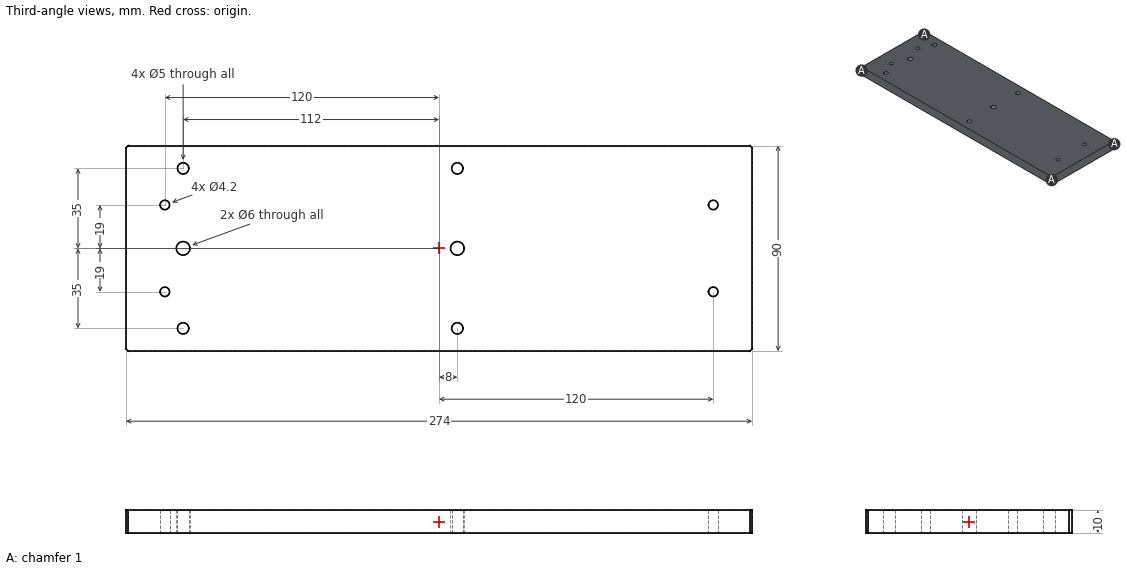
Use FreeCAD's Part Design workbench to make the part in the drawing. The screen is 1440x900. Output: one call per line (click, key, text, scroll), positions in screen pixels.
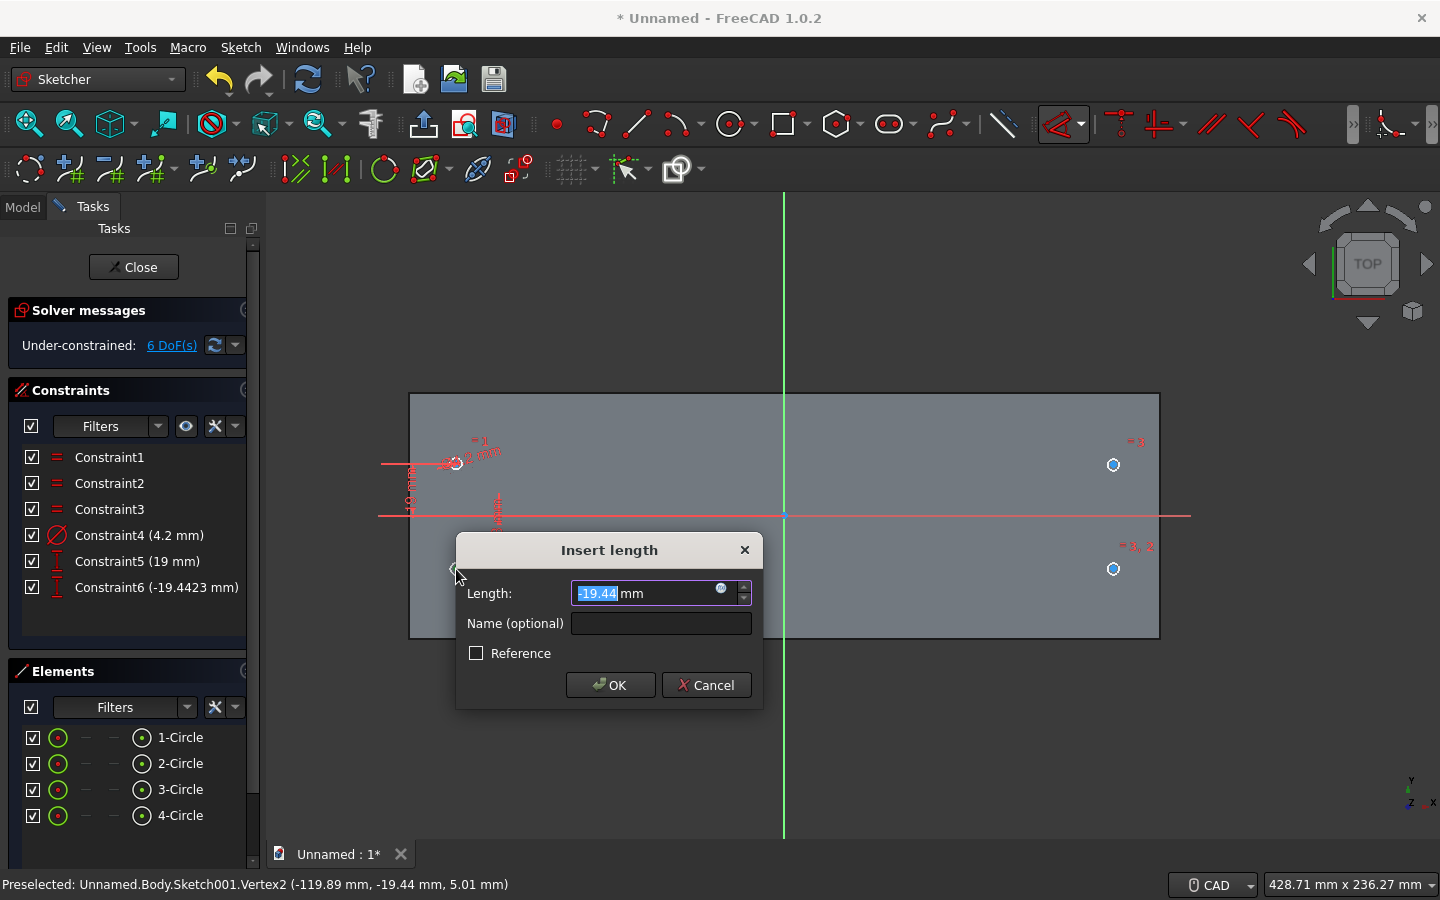
text(-19)
key(Return)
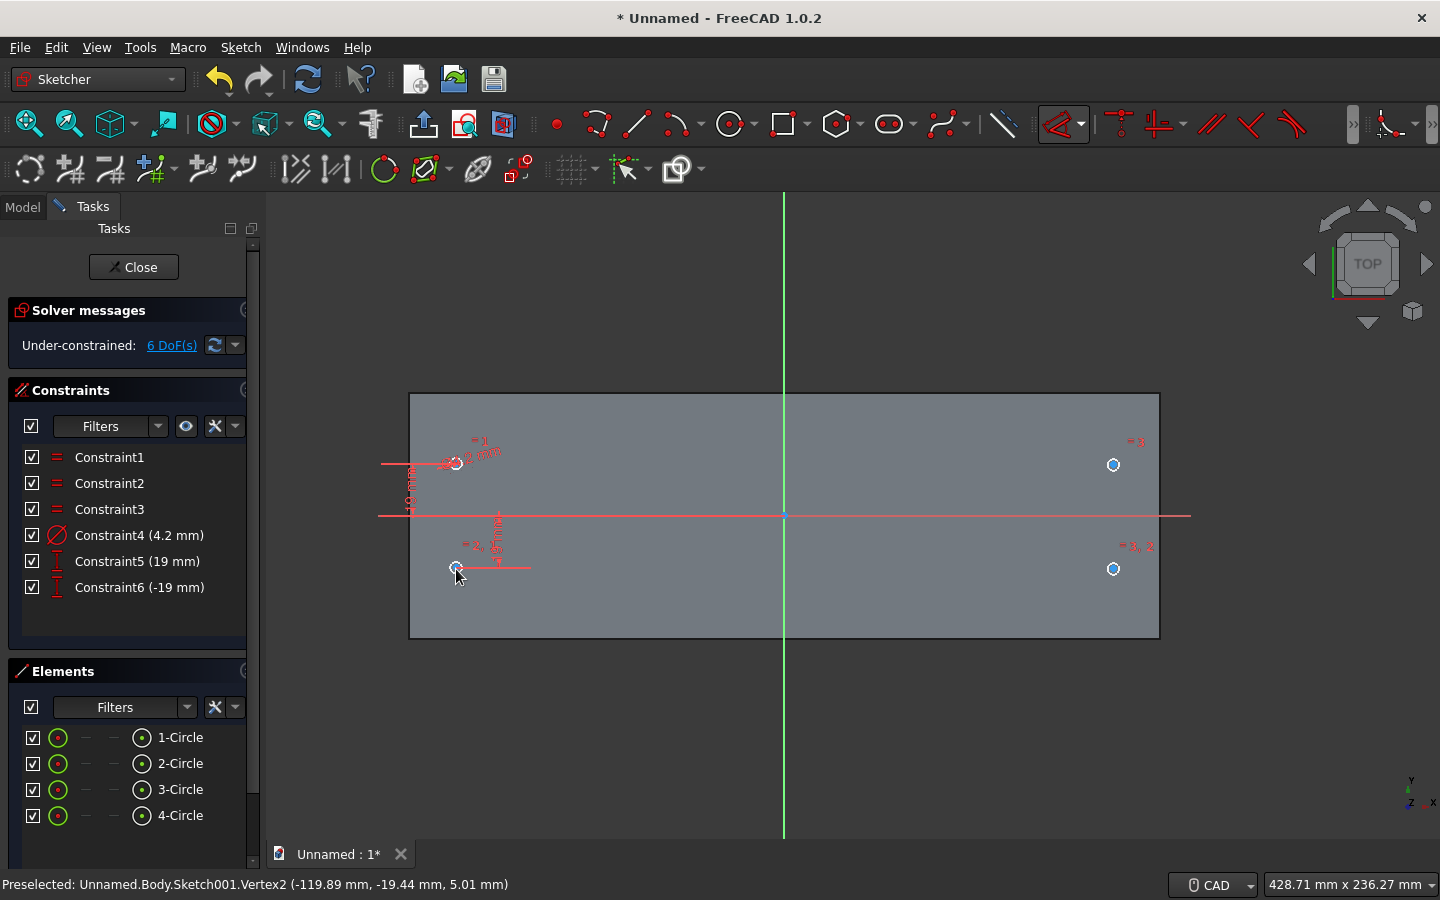
click(1113, 569)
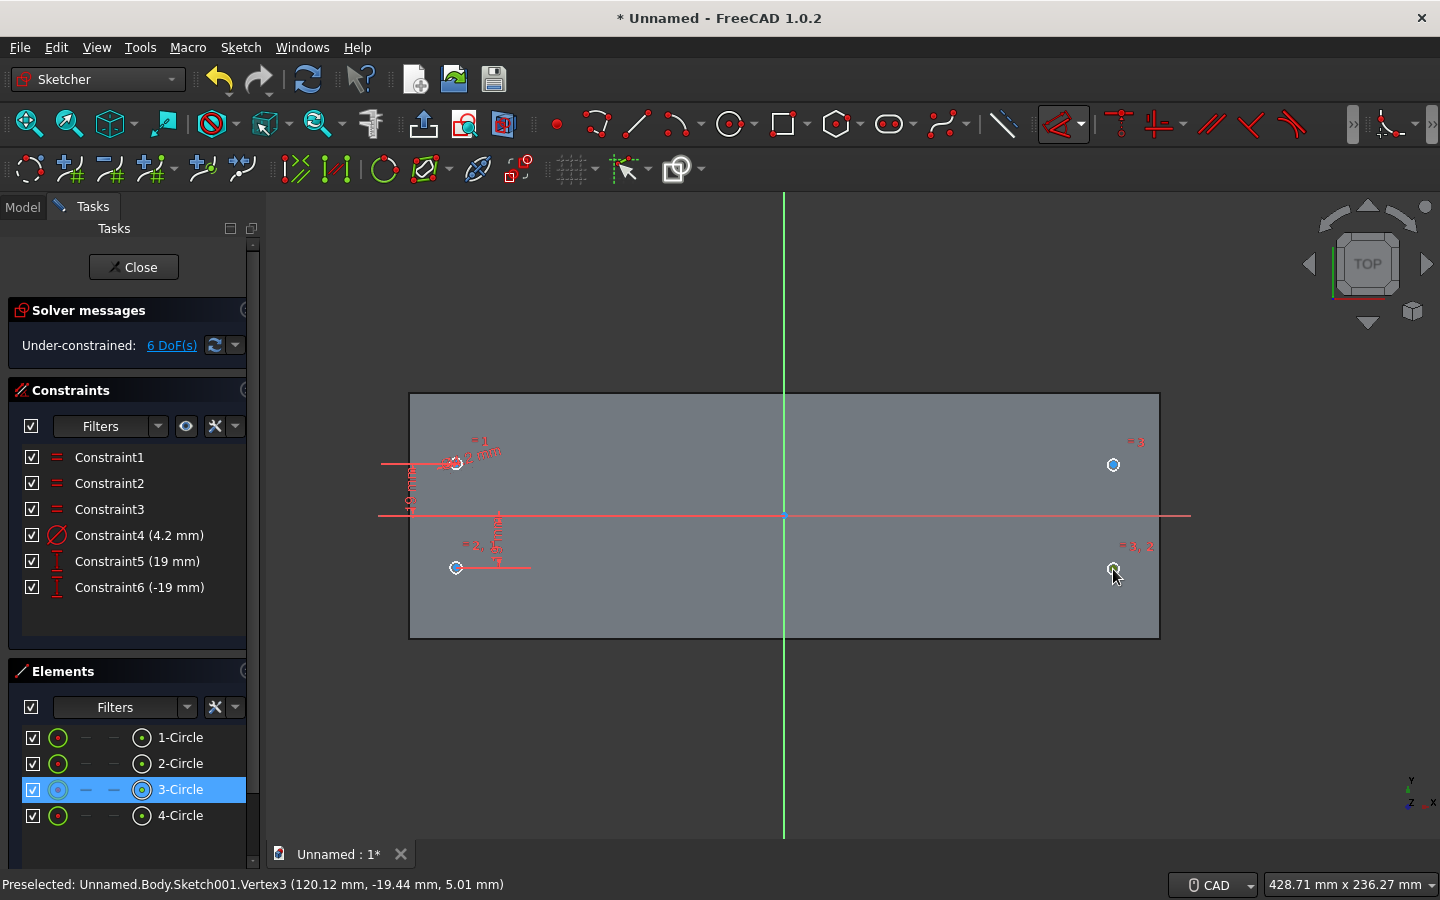
key(i)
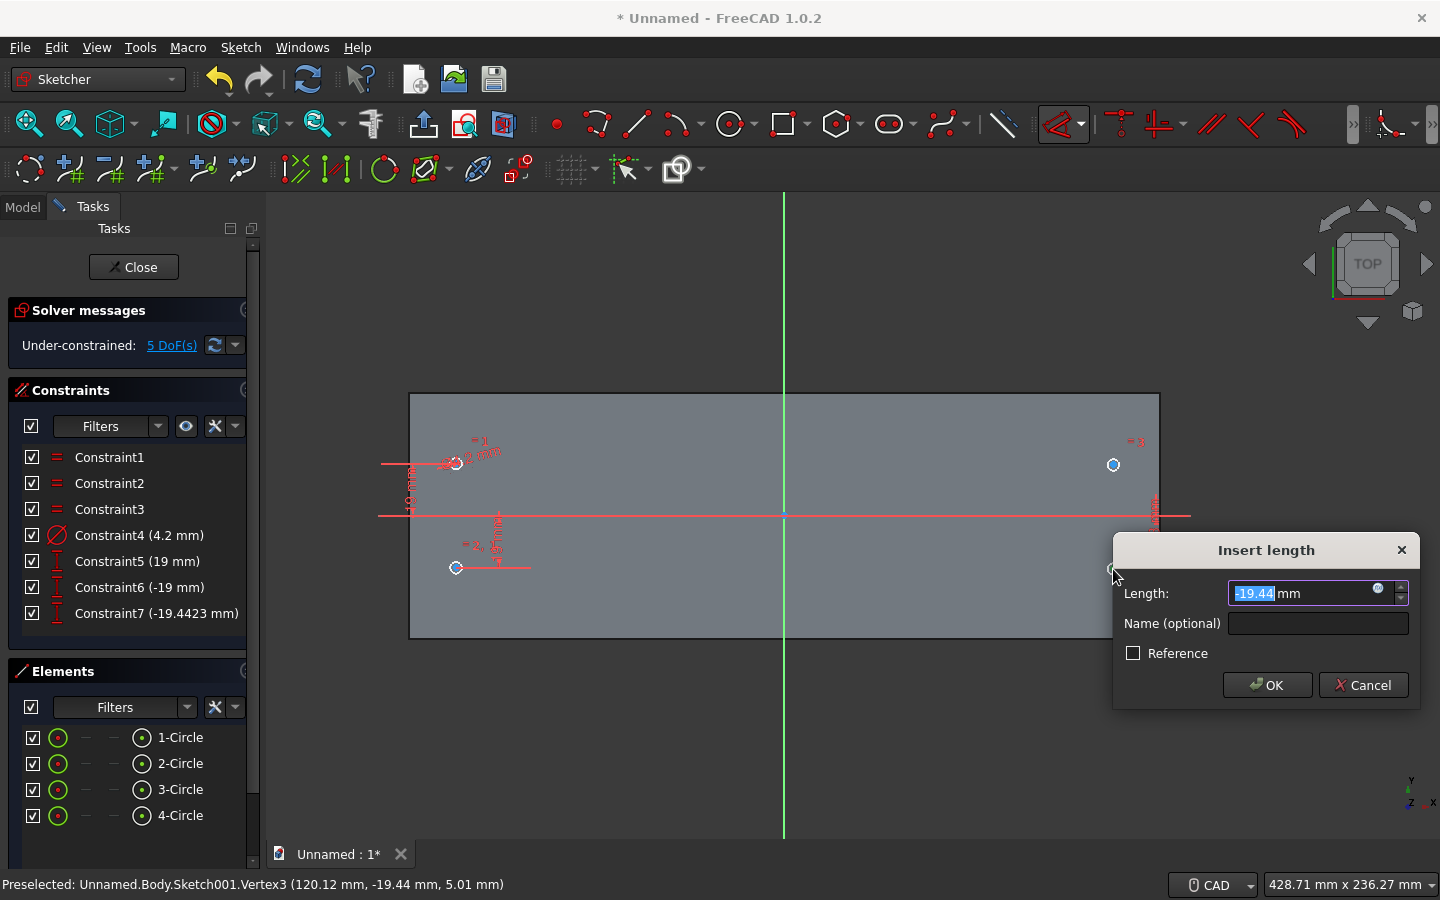
text(-19)
key(Return)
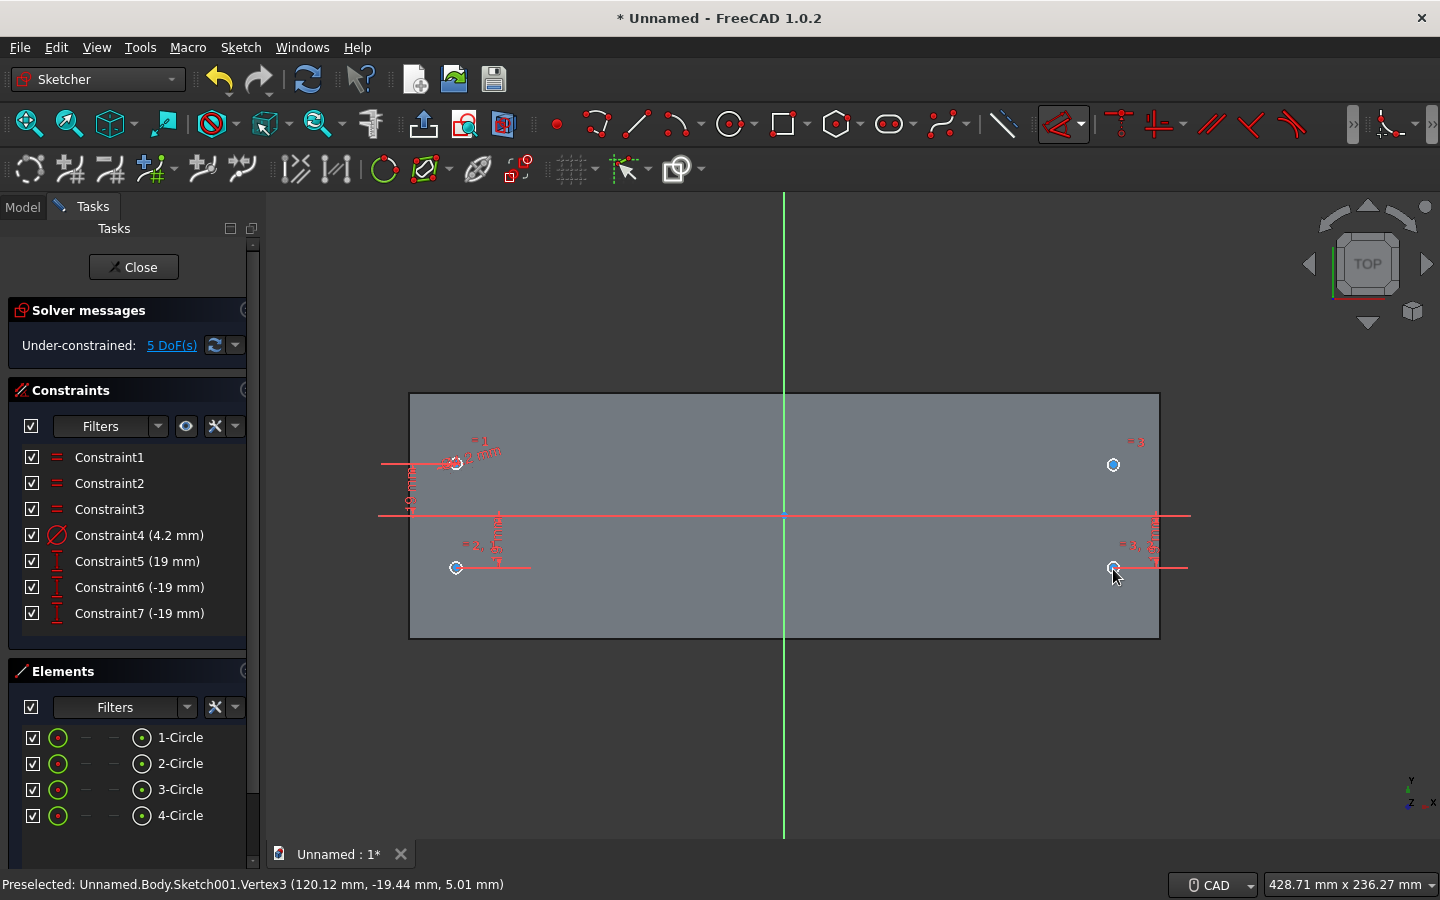
click(1113, 465)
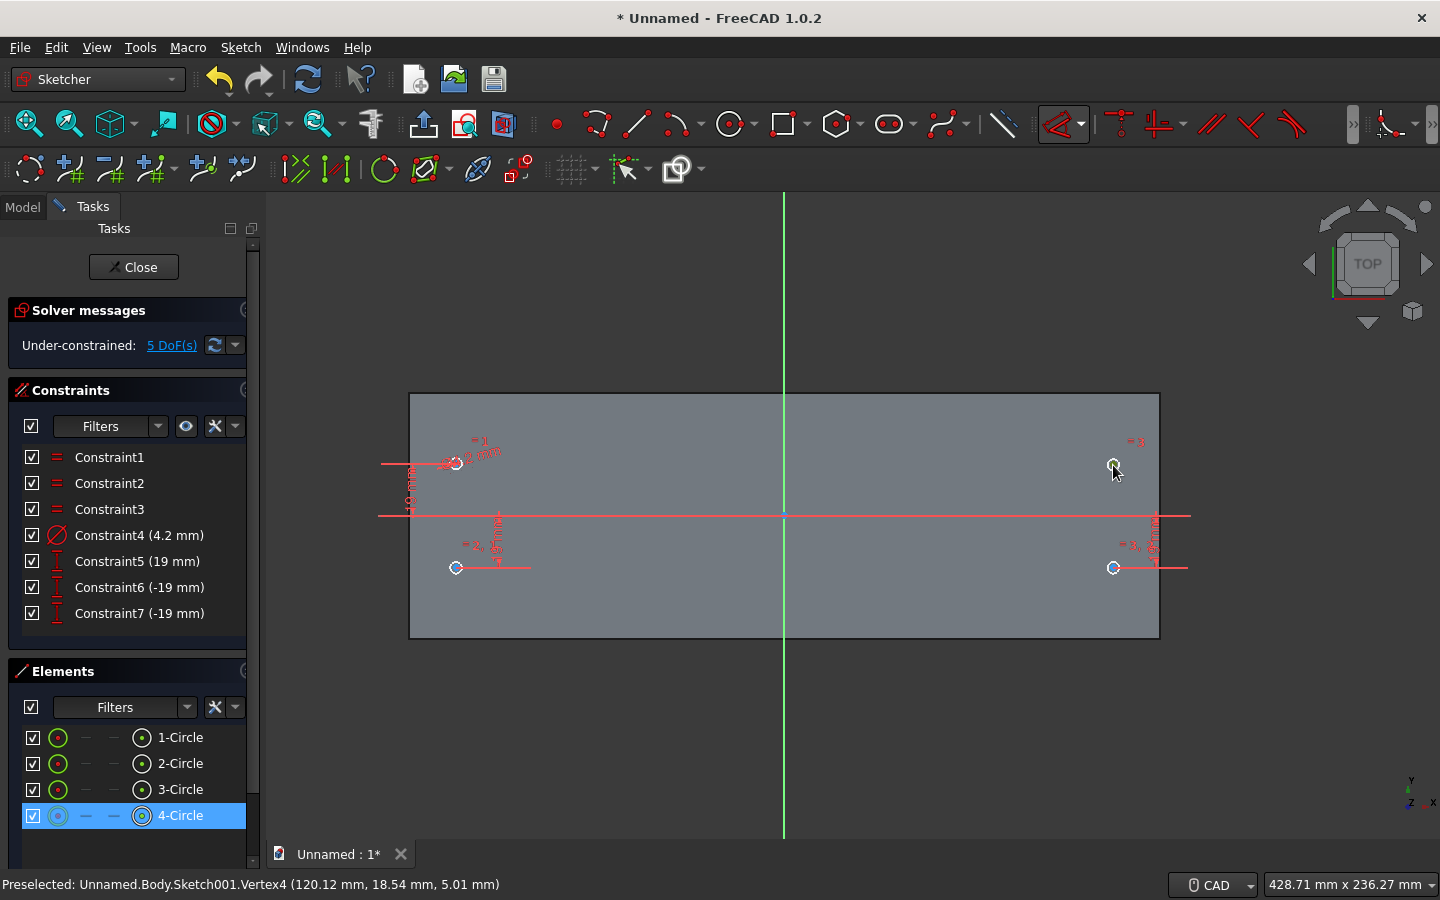
key(i)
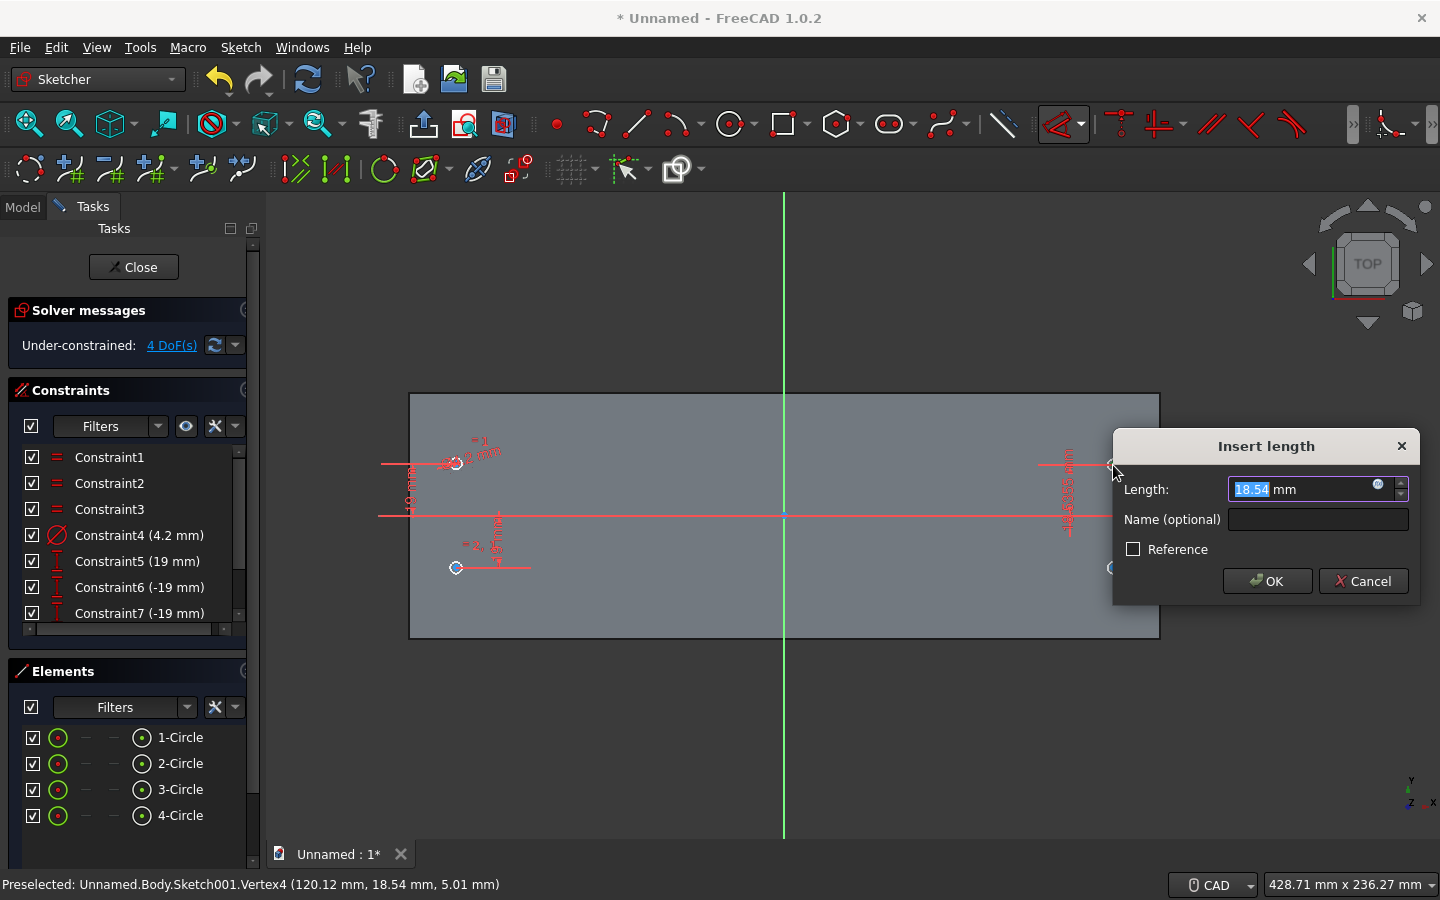
text(19)
key(Return)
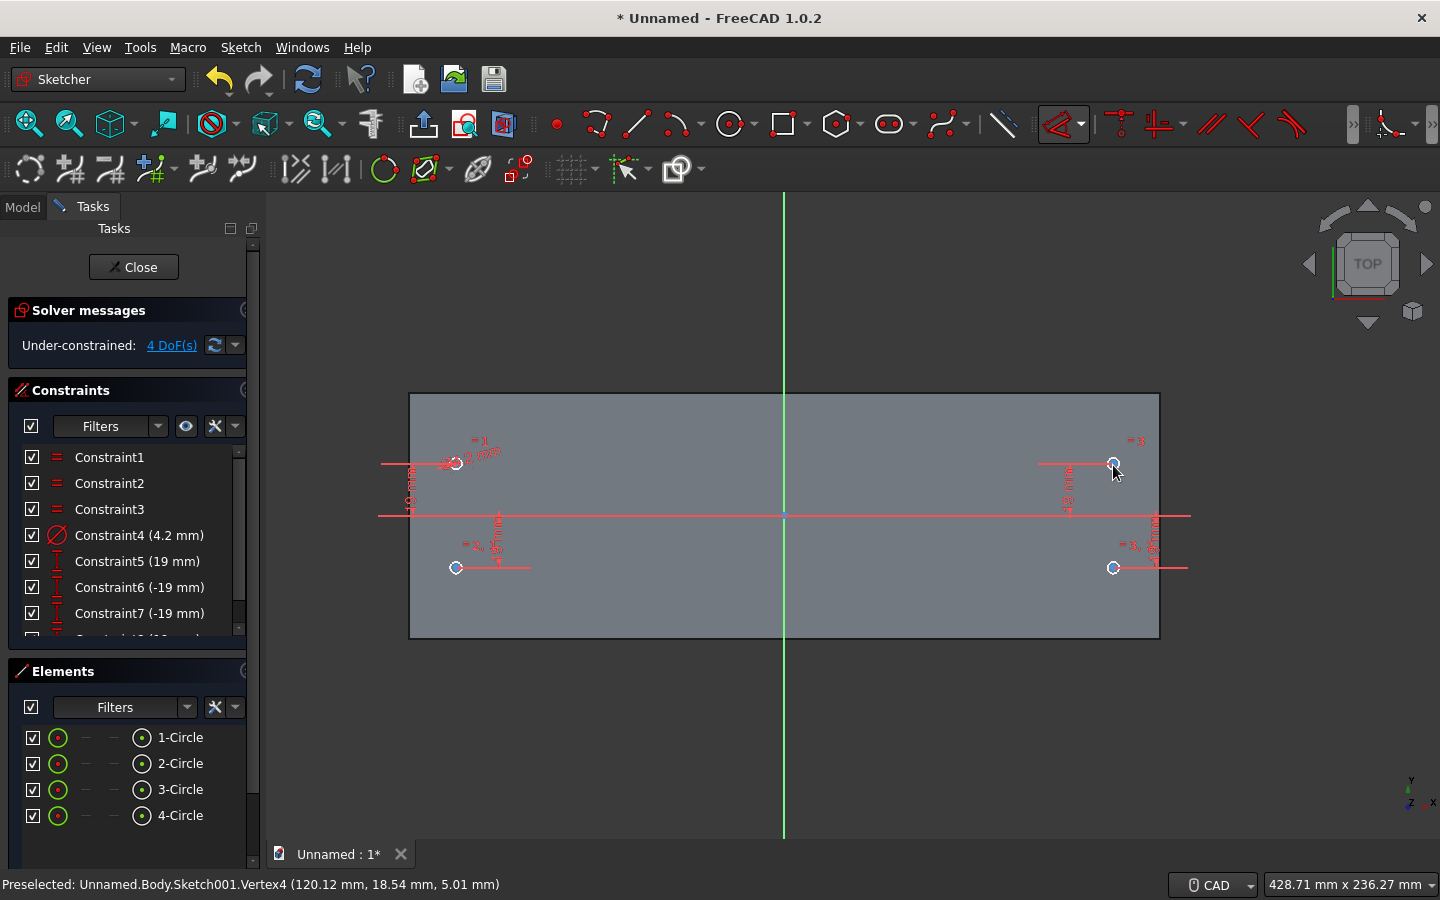
click(456, 464)